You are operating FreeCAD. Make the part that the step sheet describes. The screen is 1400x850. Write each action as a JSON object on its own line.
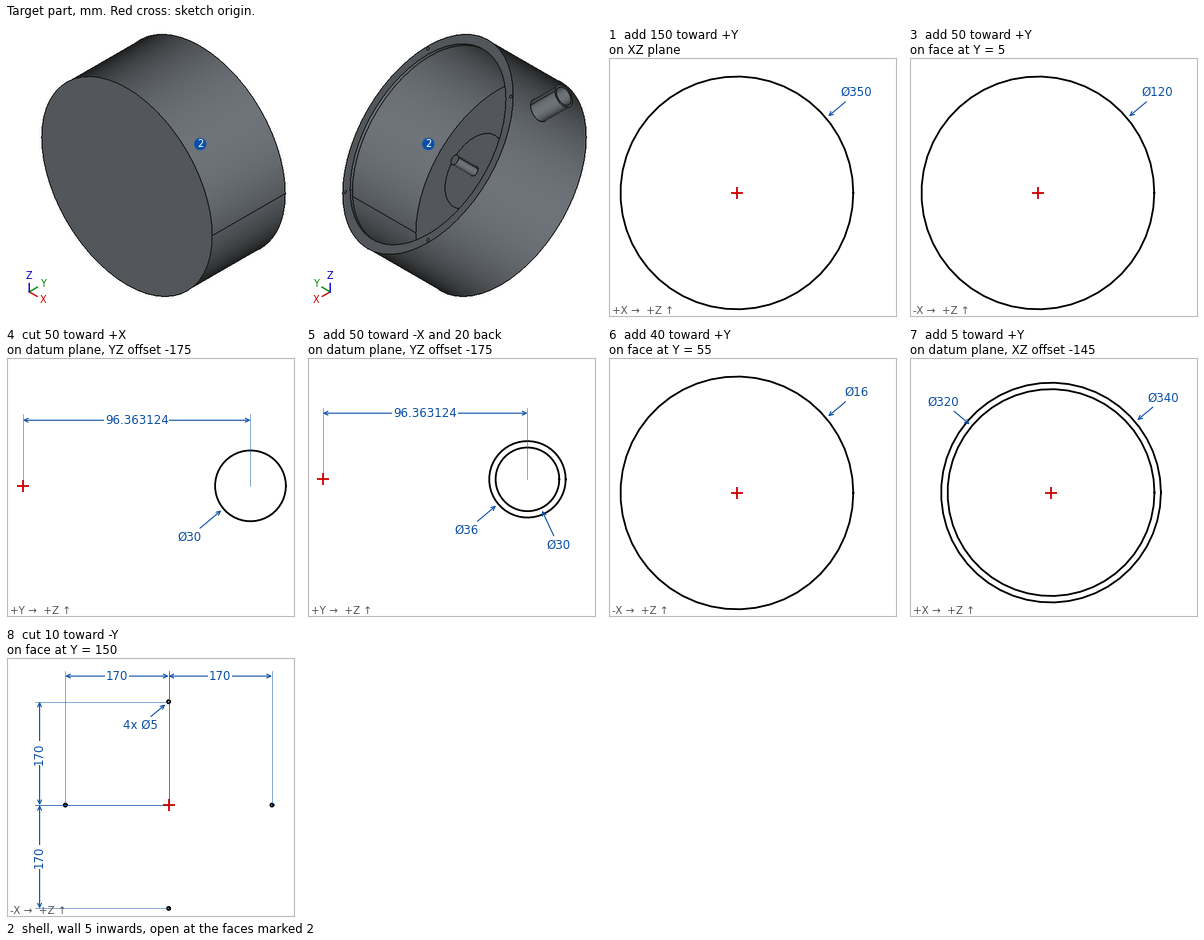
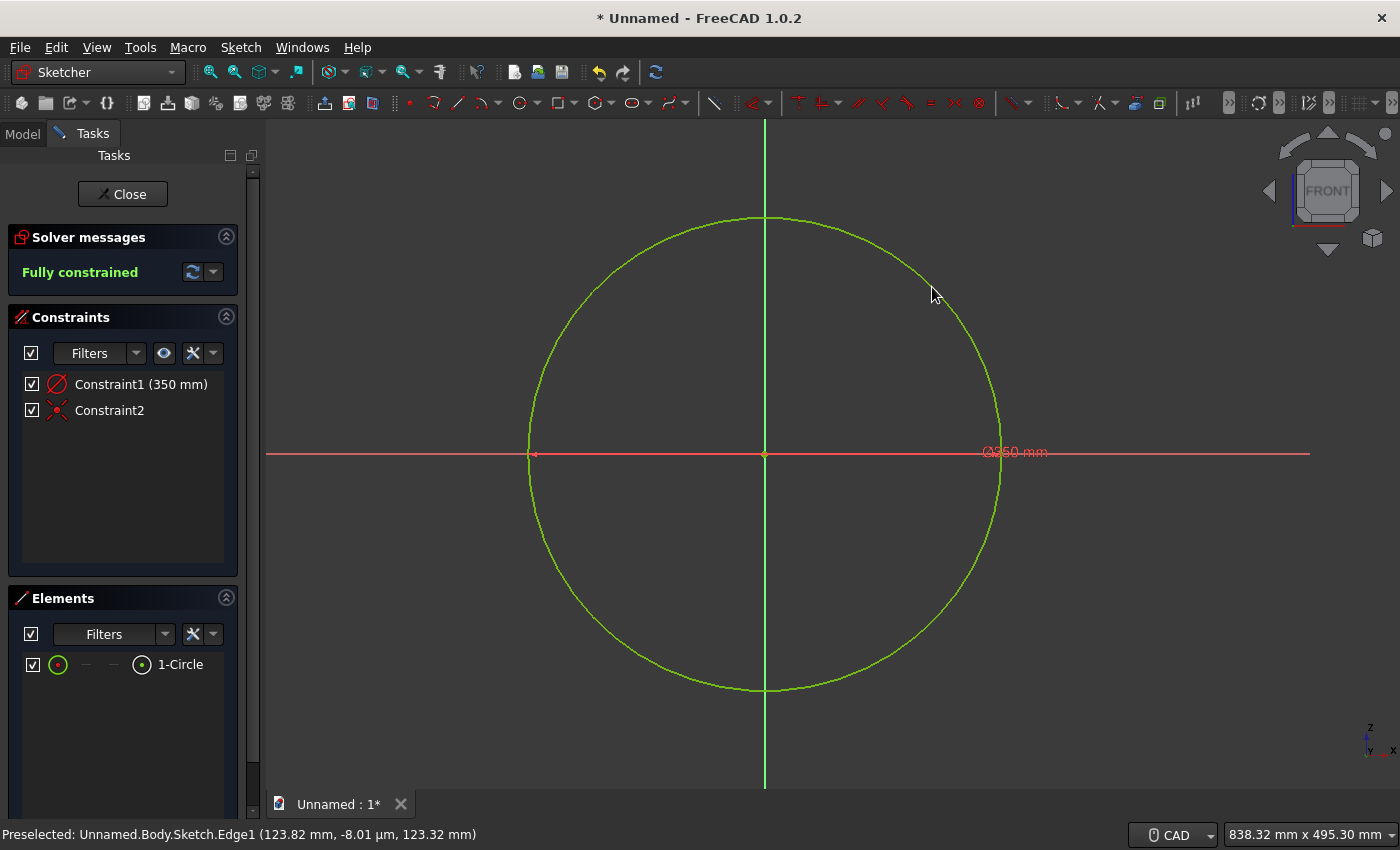
{"action": "left_click", "coordinate": [123, 194]}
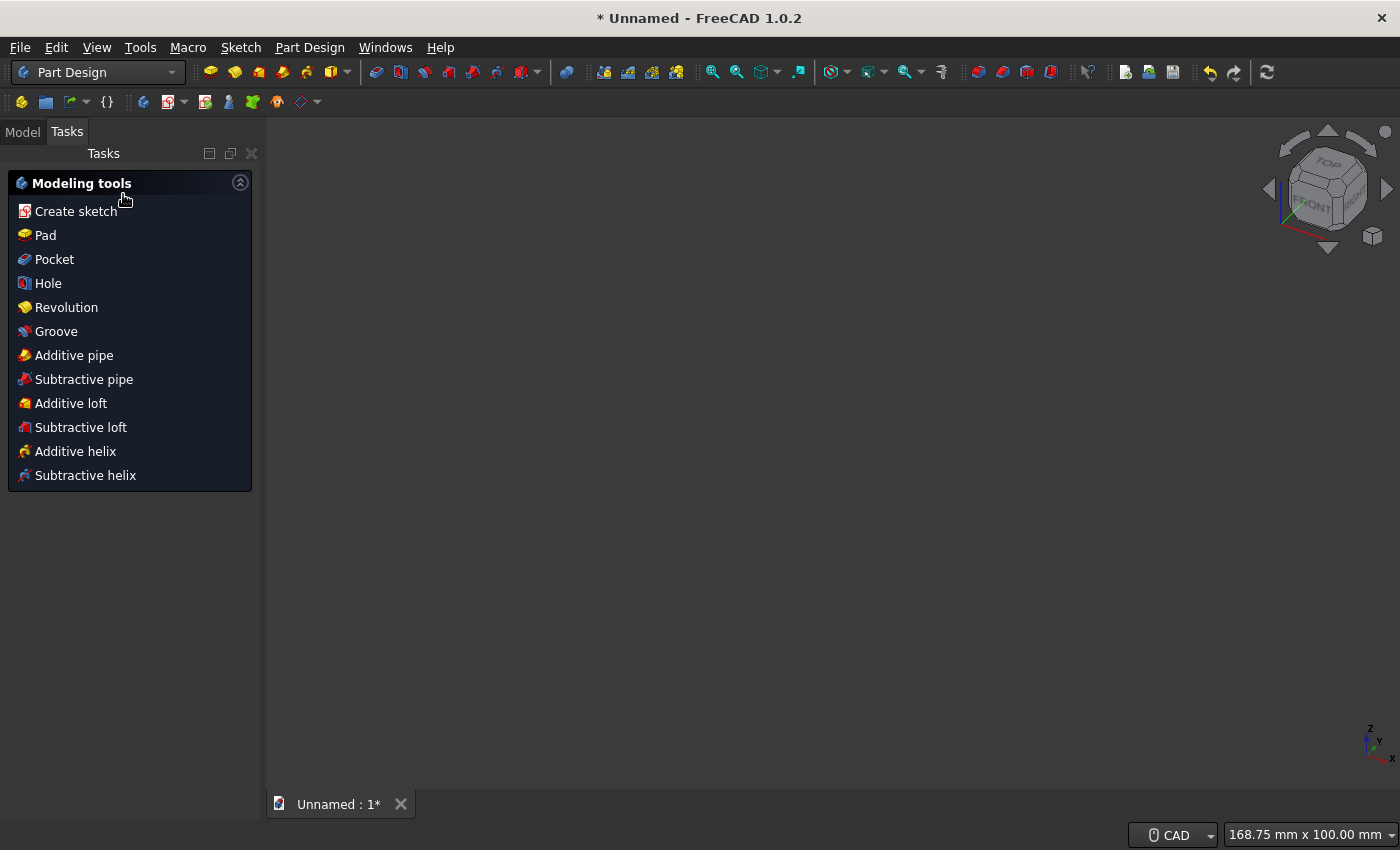
{"action": "left_click", "coordinate": [212, 72]}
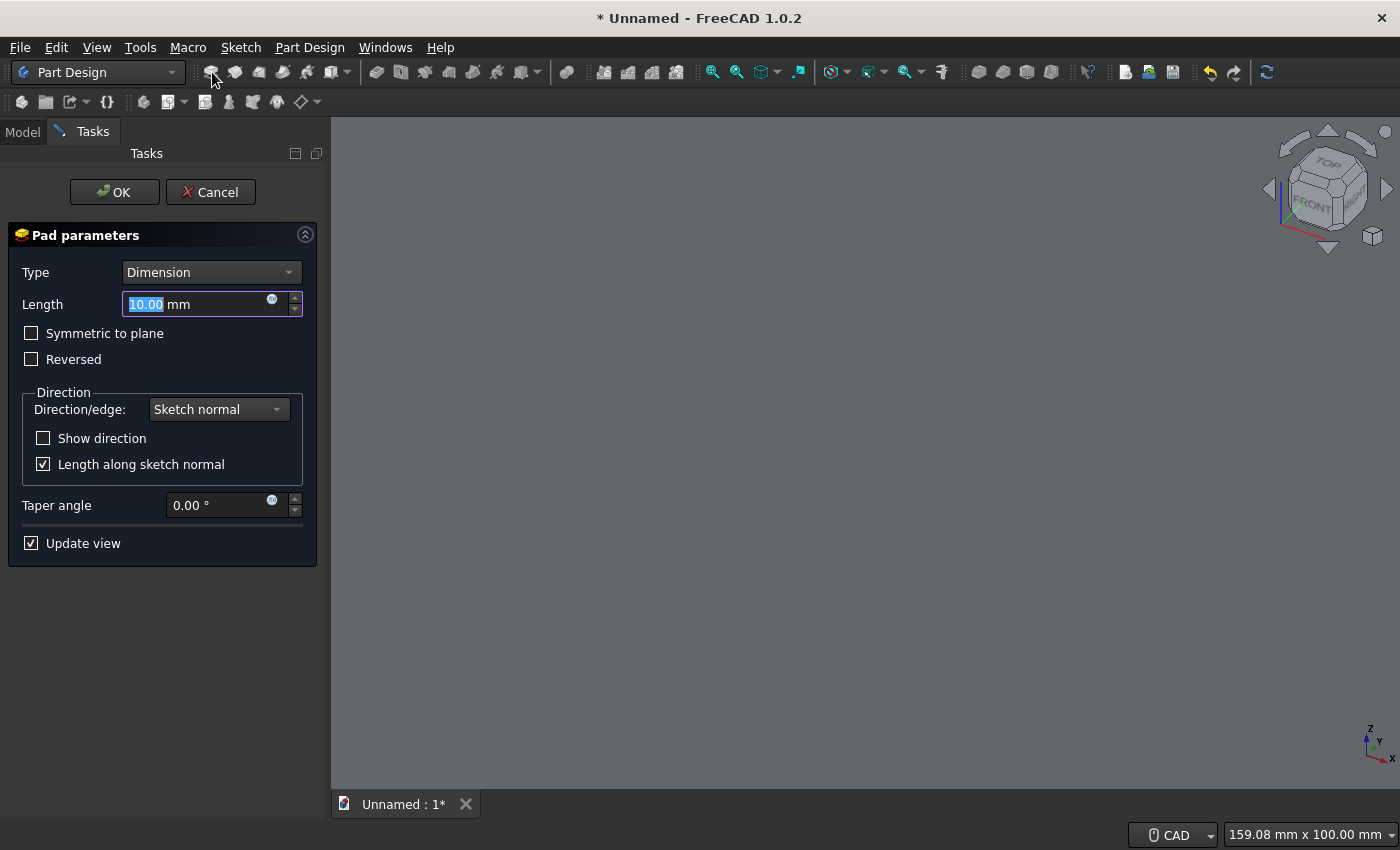
{"action": "type", "text": "150"}
{"action": "key", "text": "Tab"}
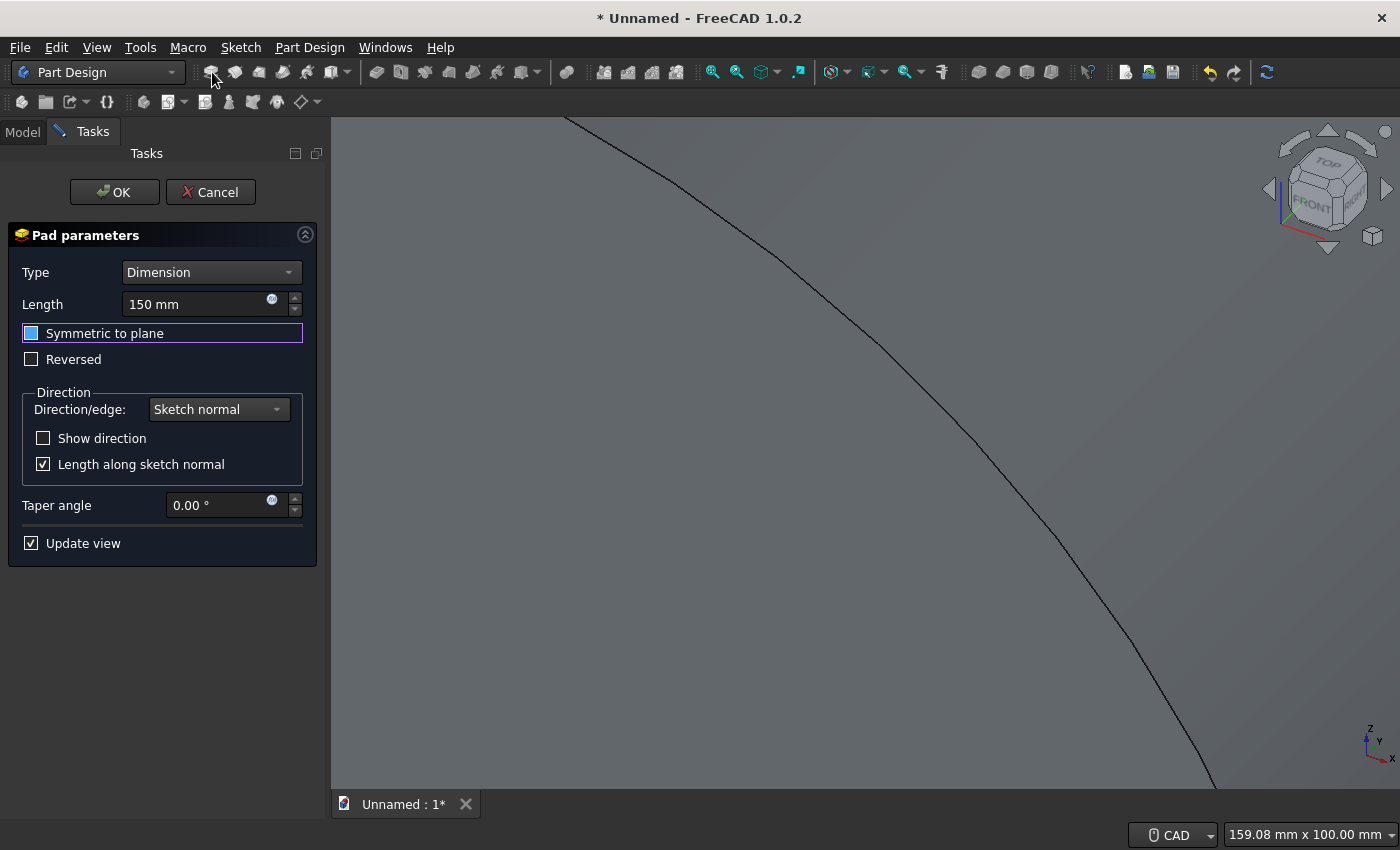
{"action": "left_click", "coordinate": [30, 359]}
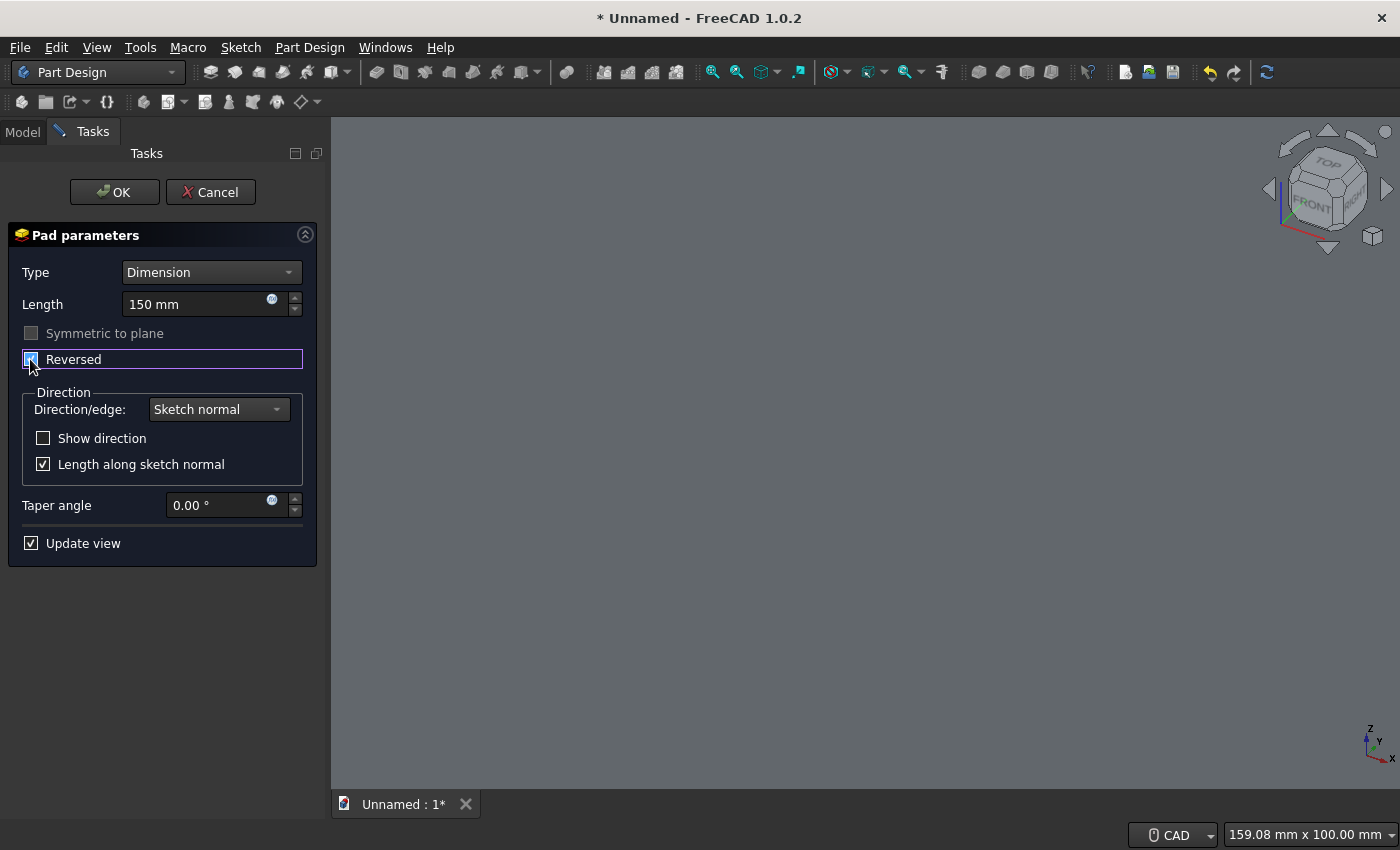
{"action": "left_click", "coordinate": [115, 192]}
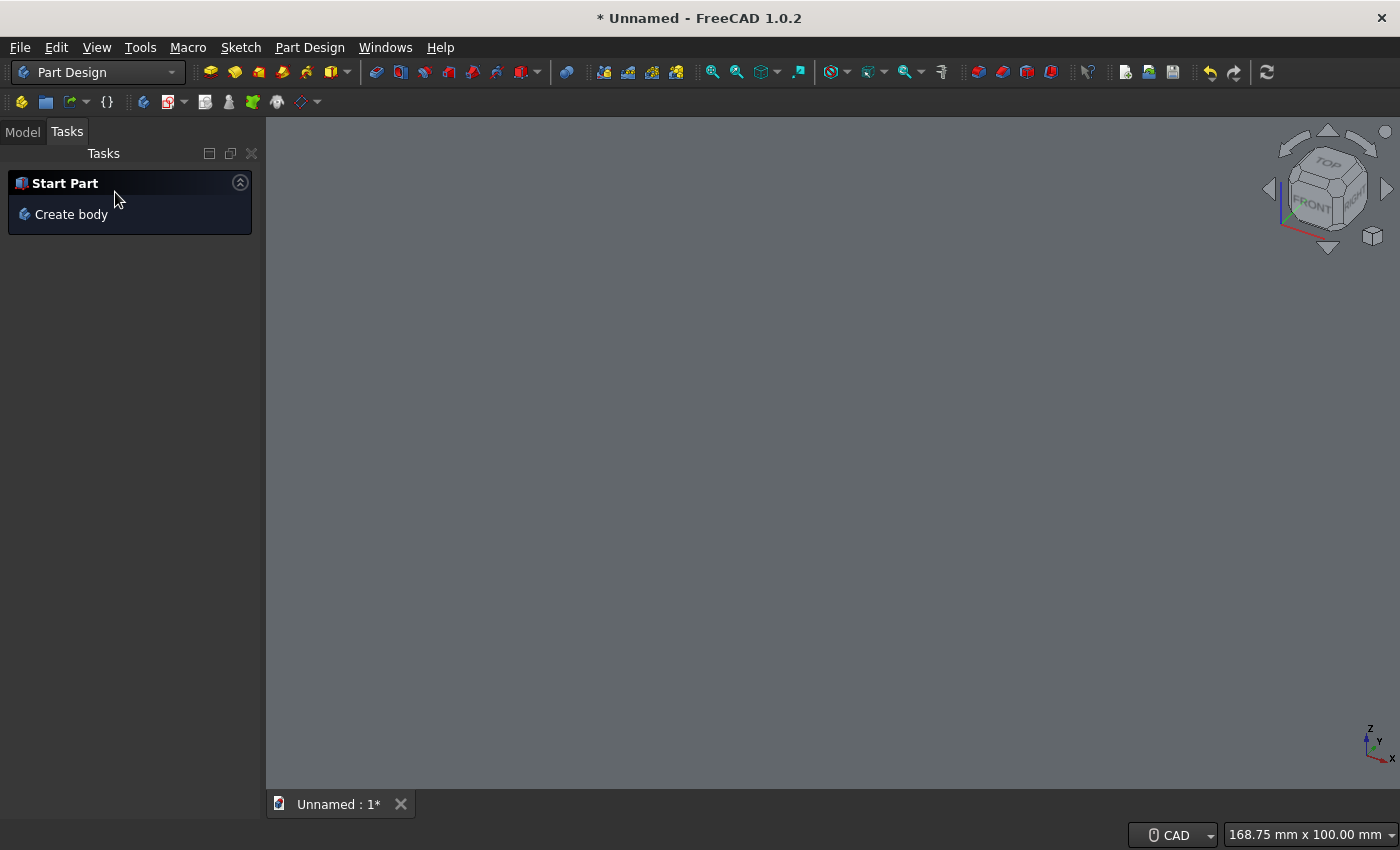
{"action": "left_click", "coordinate": [714, 72]}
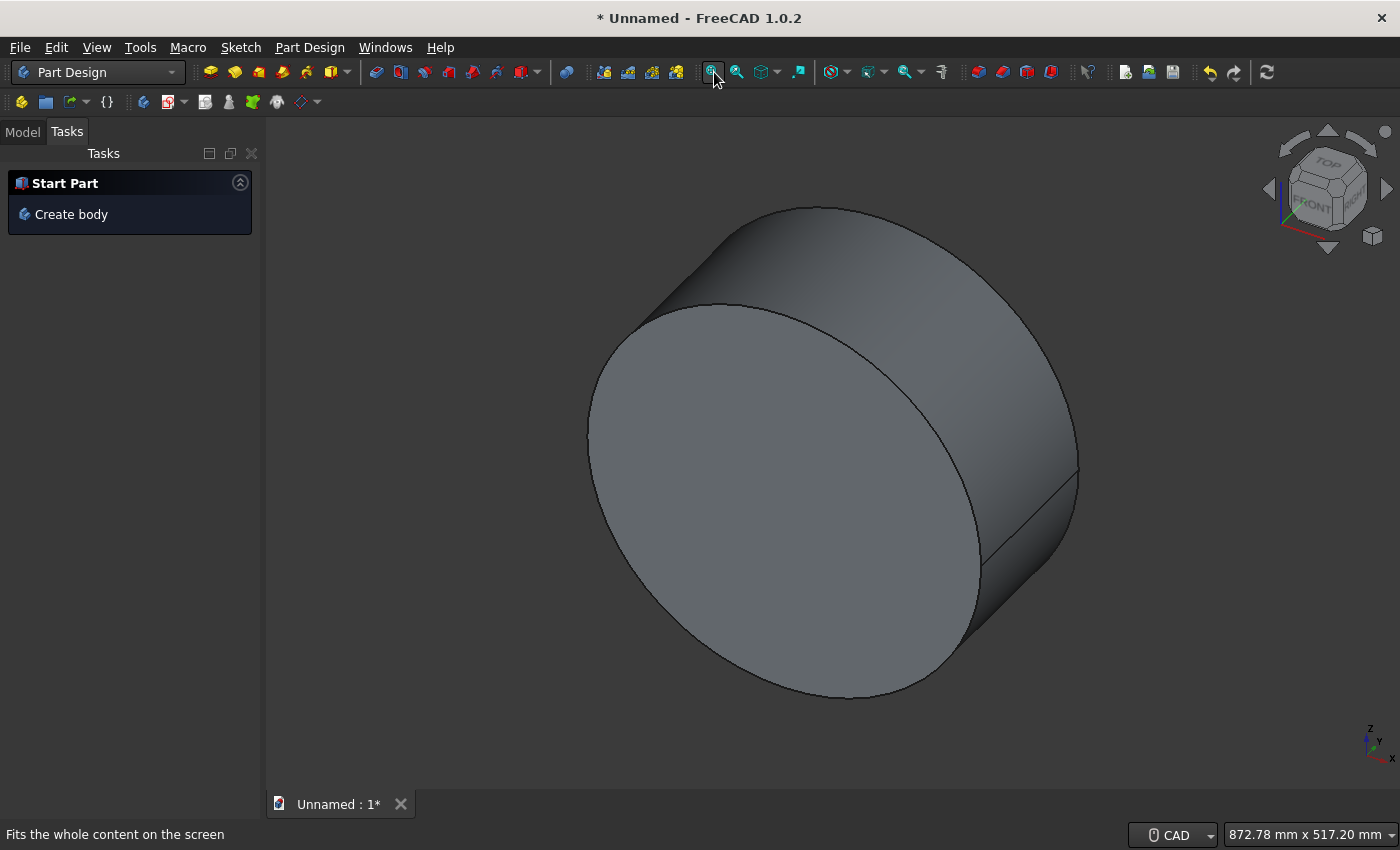
{"action": "key", "text": "0"}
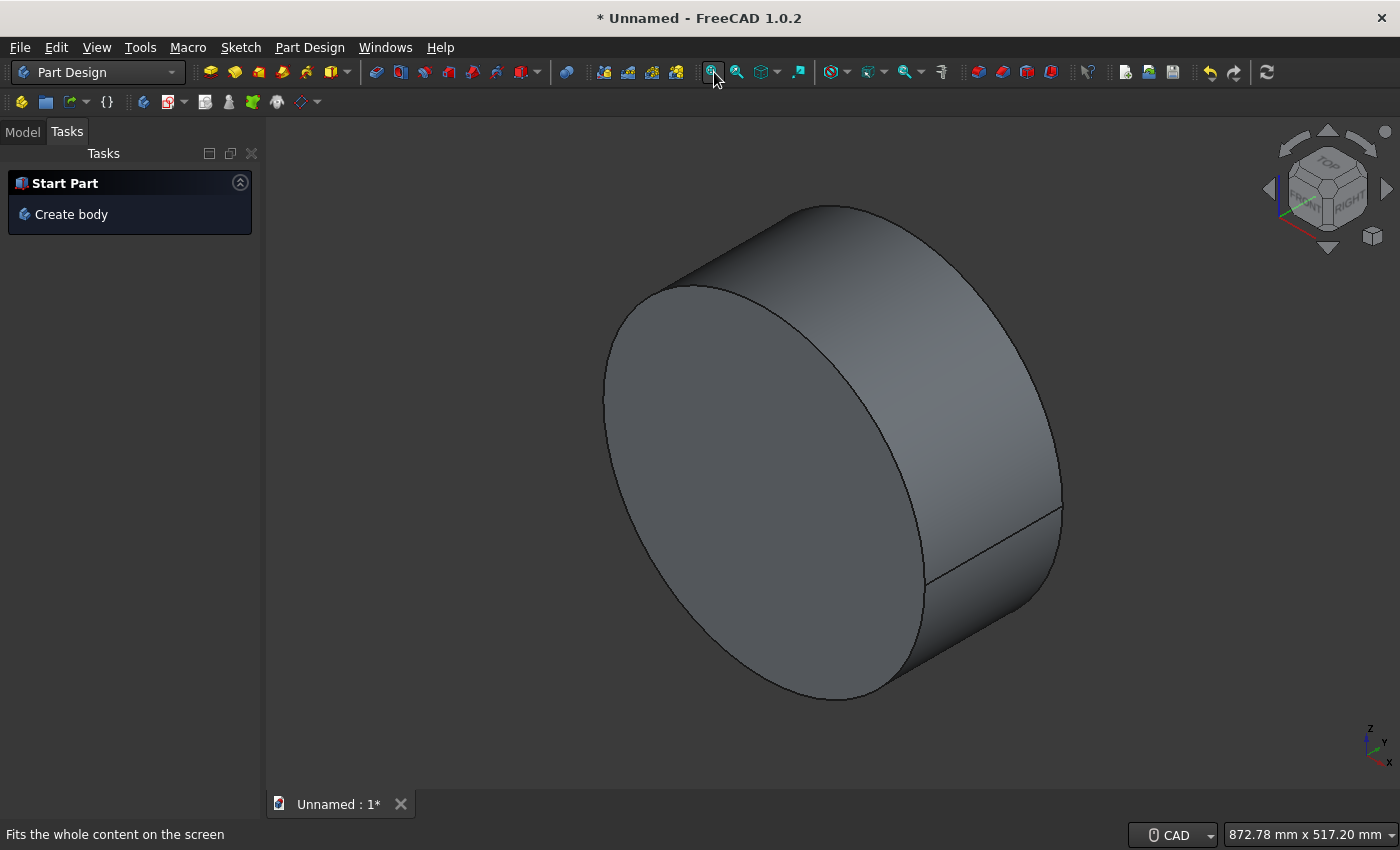
{"action": "key", "text": "2"}